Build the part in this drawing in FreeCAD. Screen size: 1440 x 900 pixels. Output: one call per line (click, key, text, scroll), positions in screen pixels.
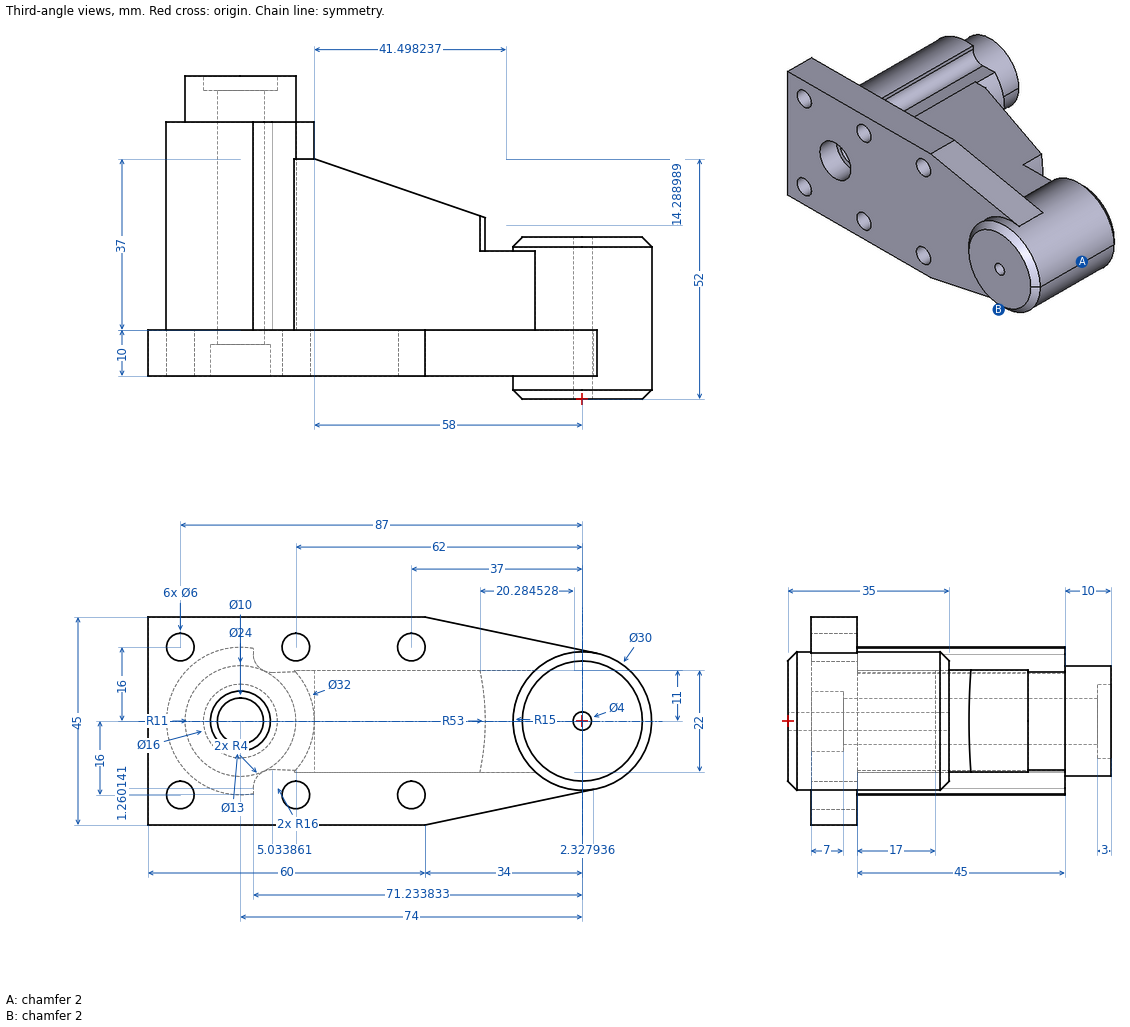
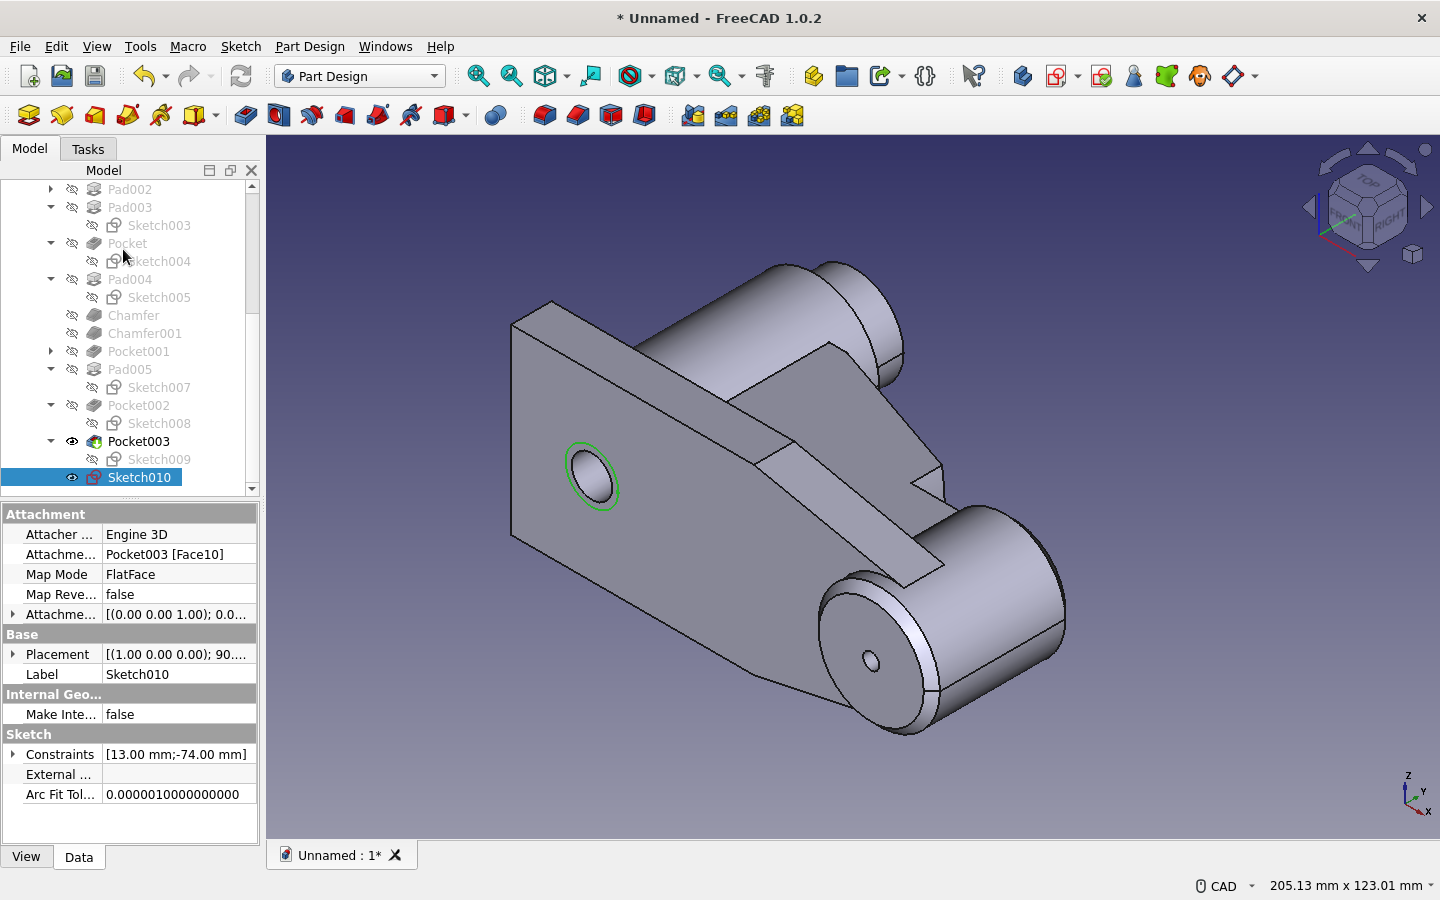
click(246, 116)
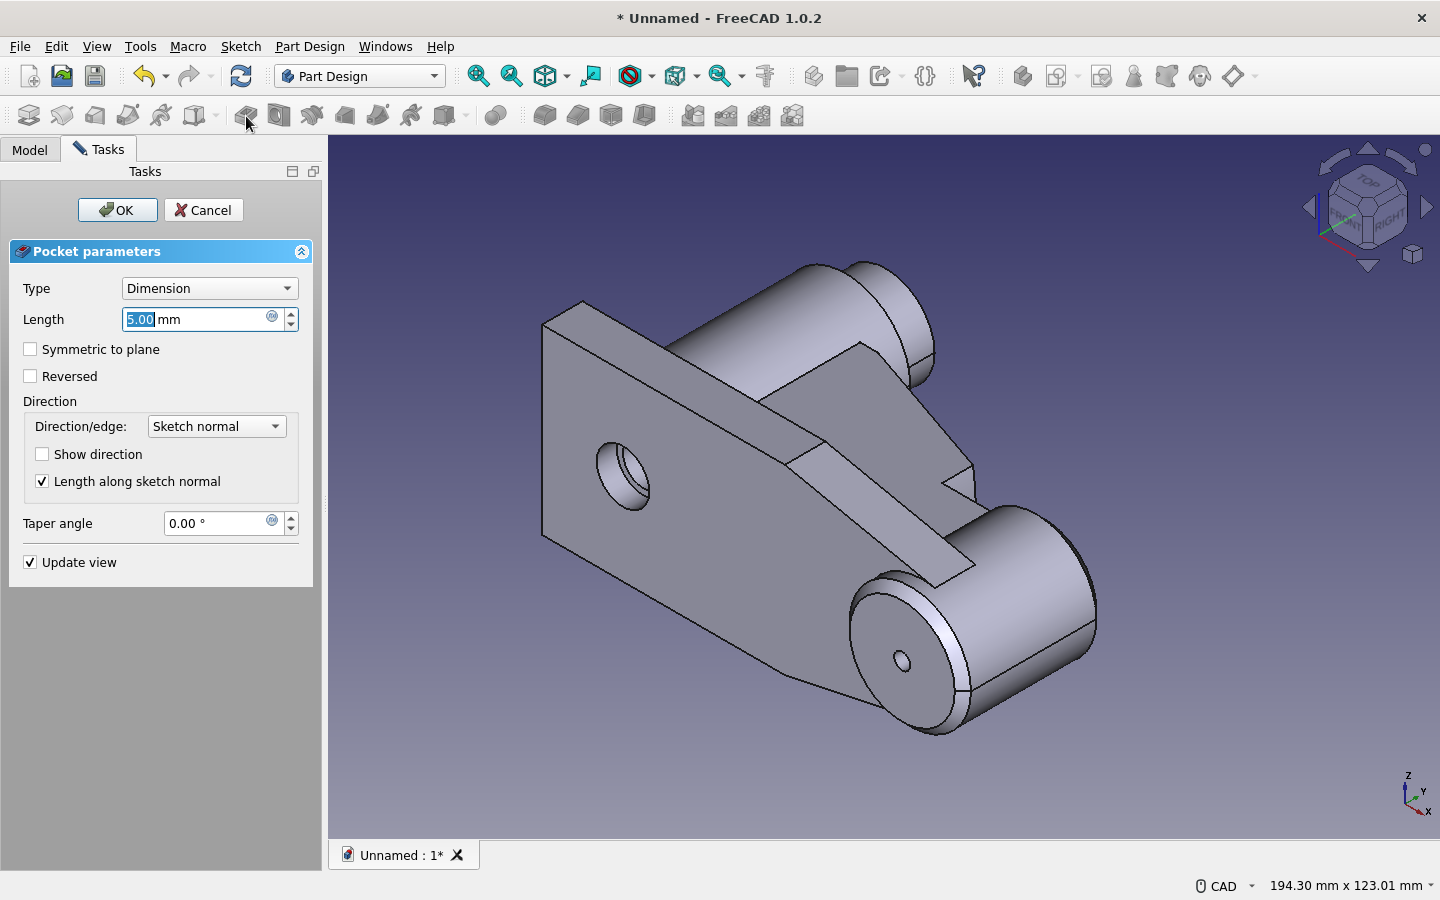
text(7)
key(Tab)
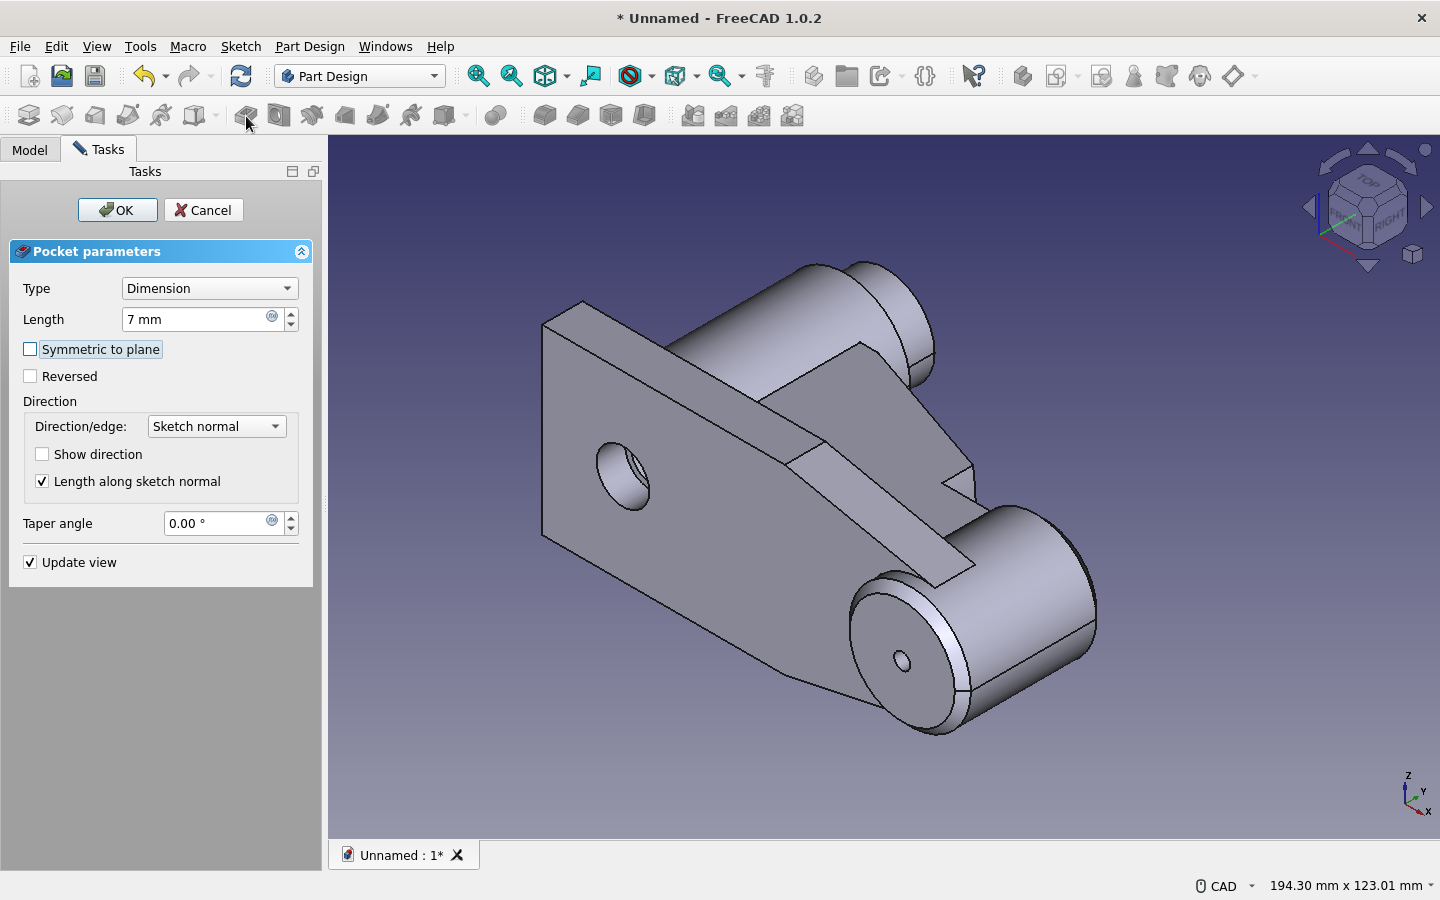
click(118, 210)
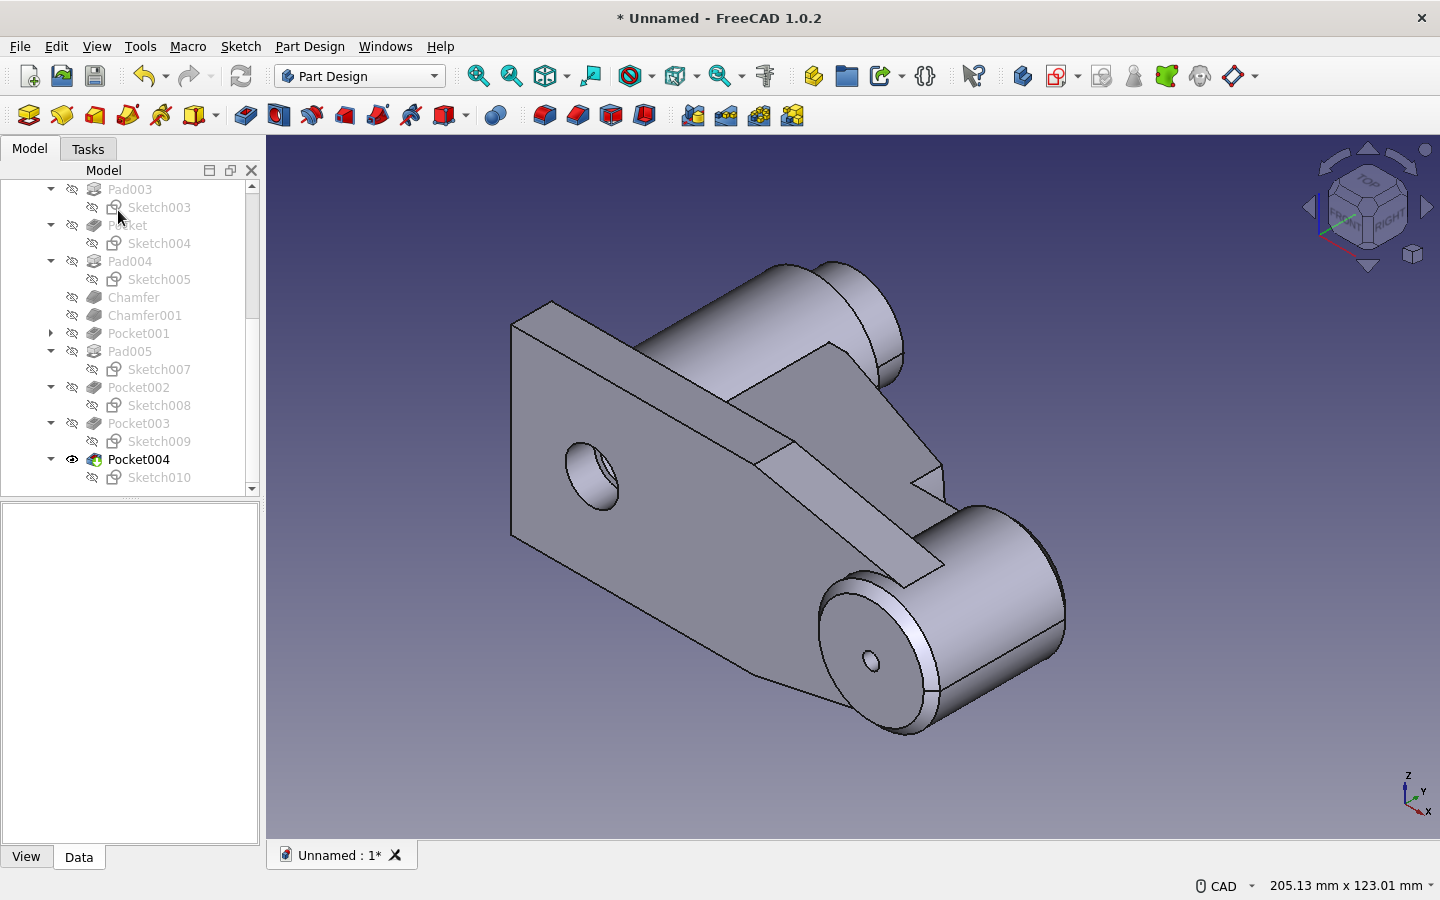
key(4)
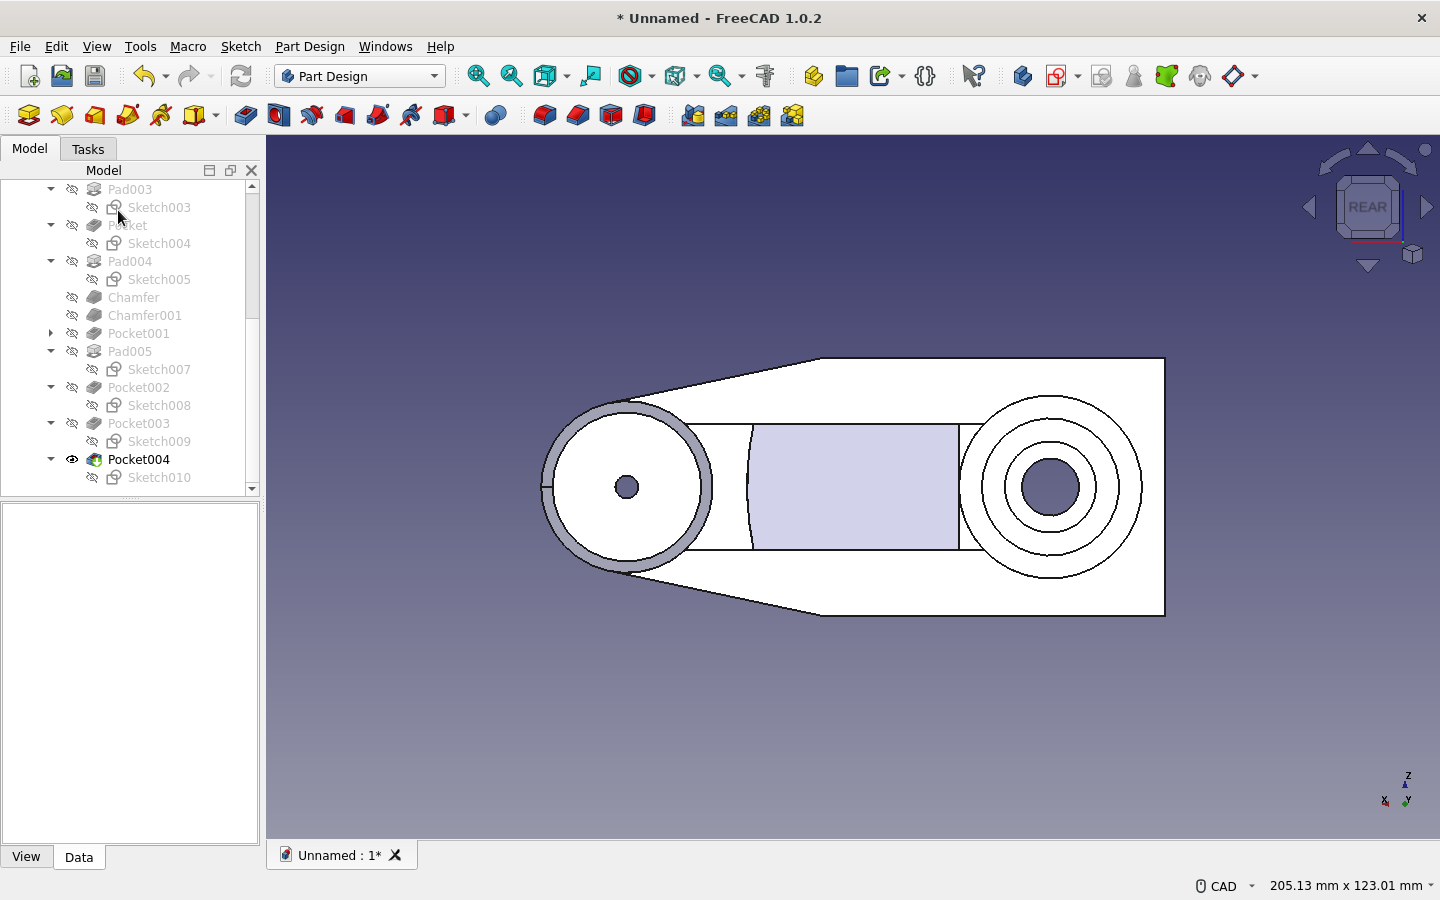
click(887, 376)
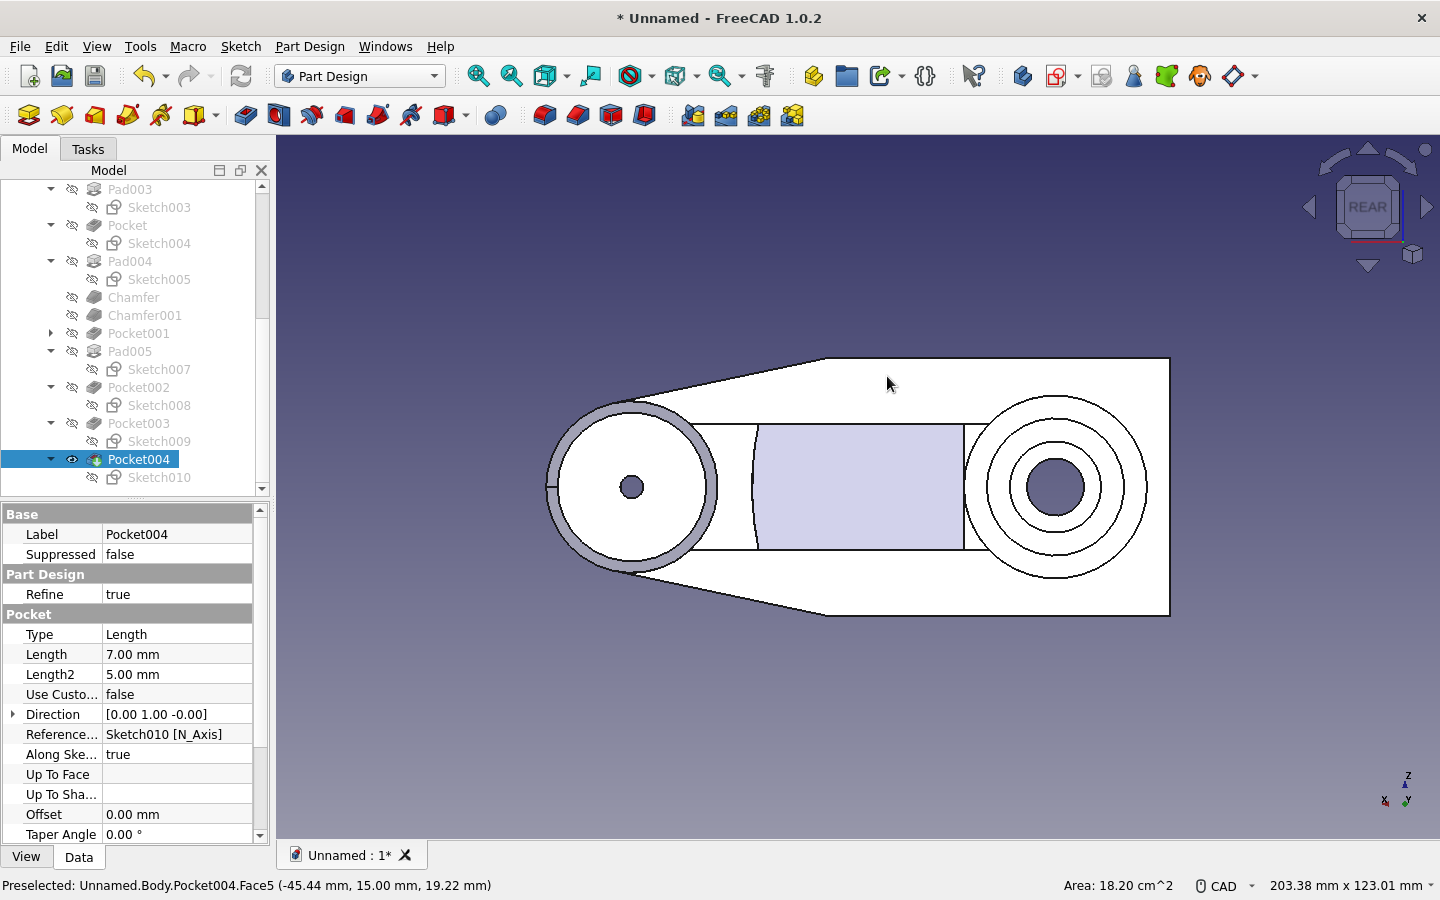
click(1056, 76)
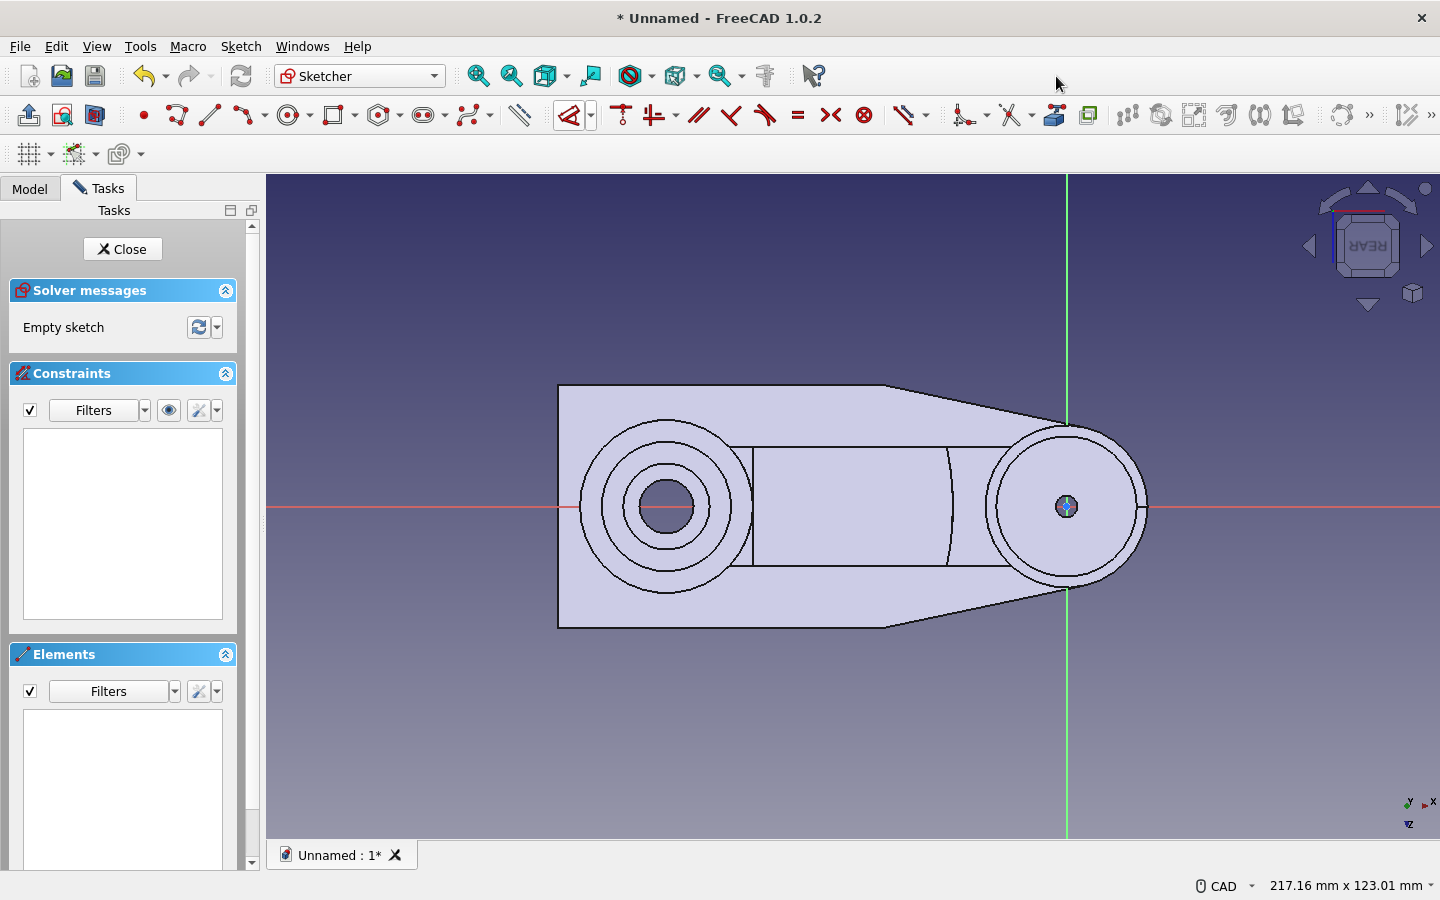
click(95, 116)